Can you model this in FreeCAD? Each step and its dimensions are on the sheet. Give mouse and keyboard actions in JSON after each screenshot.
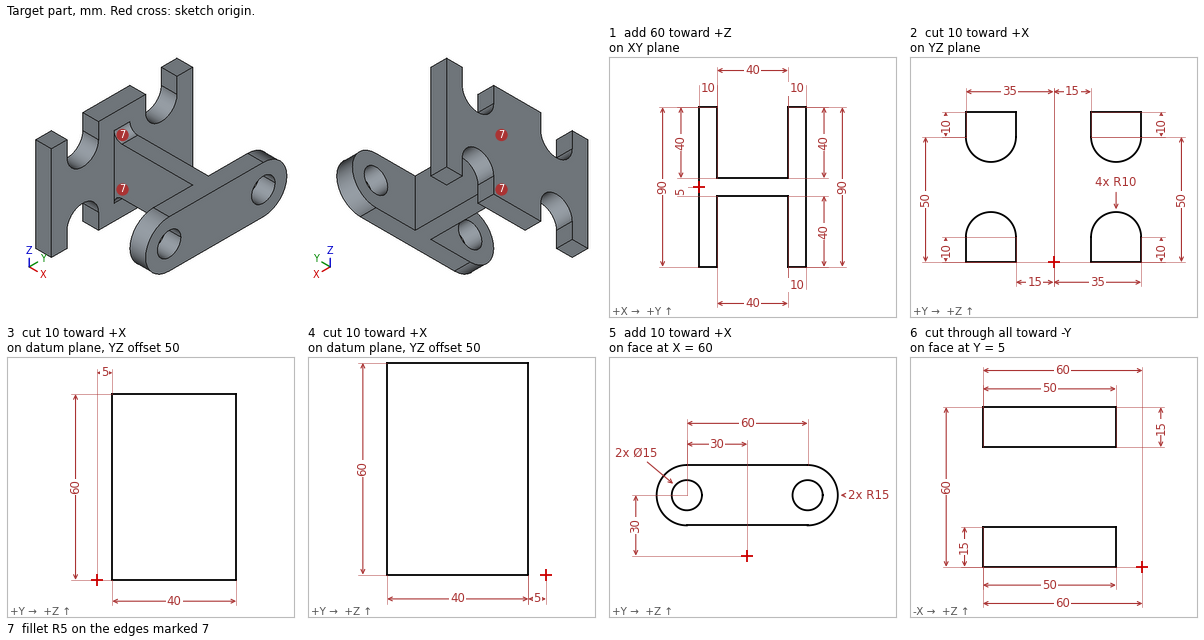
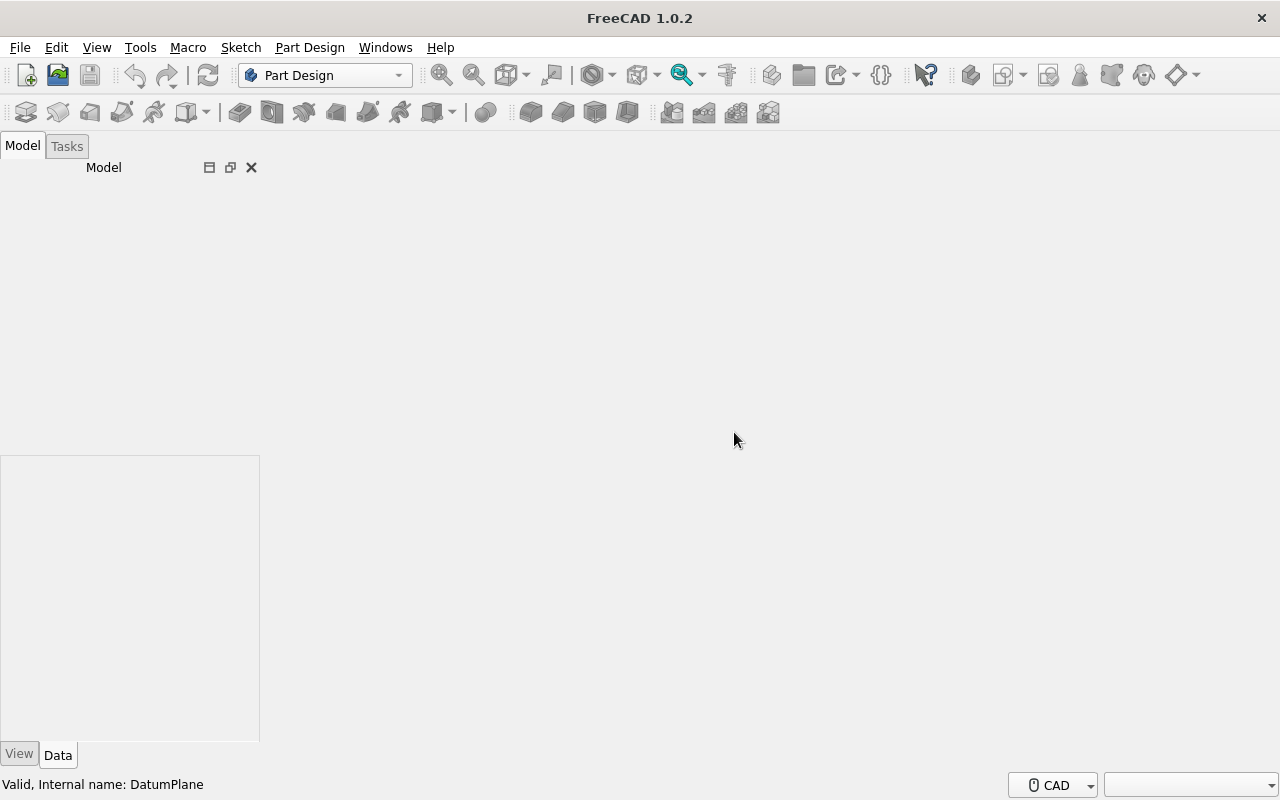
{"action": "left_click", "coordinate": [26, 76]}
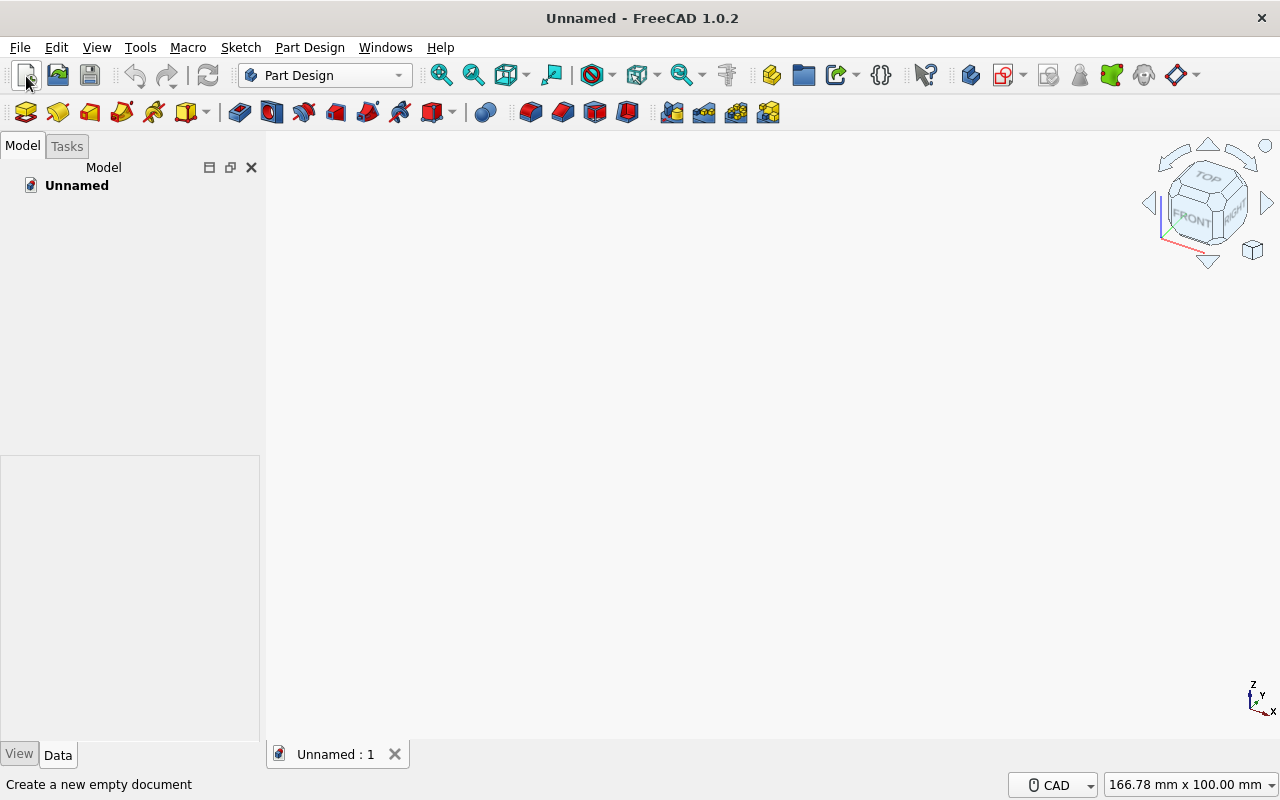
{"action": "left_click", "coordinate": [1004, 76]}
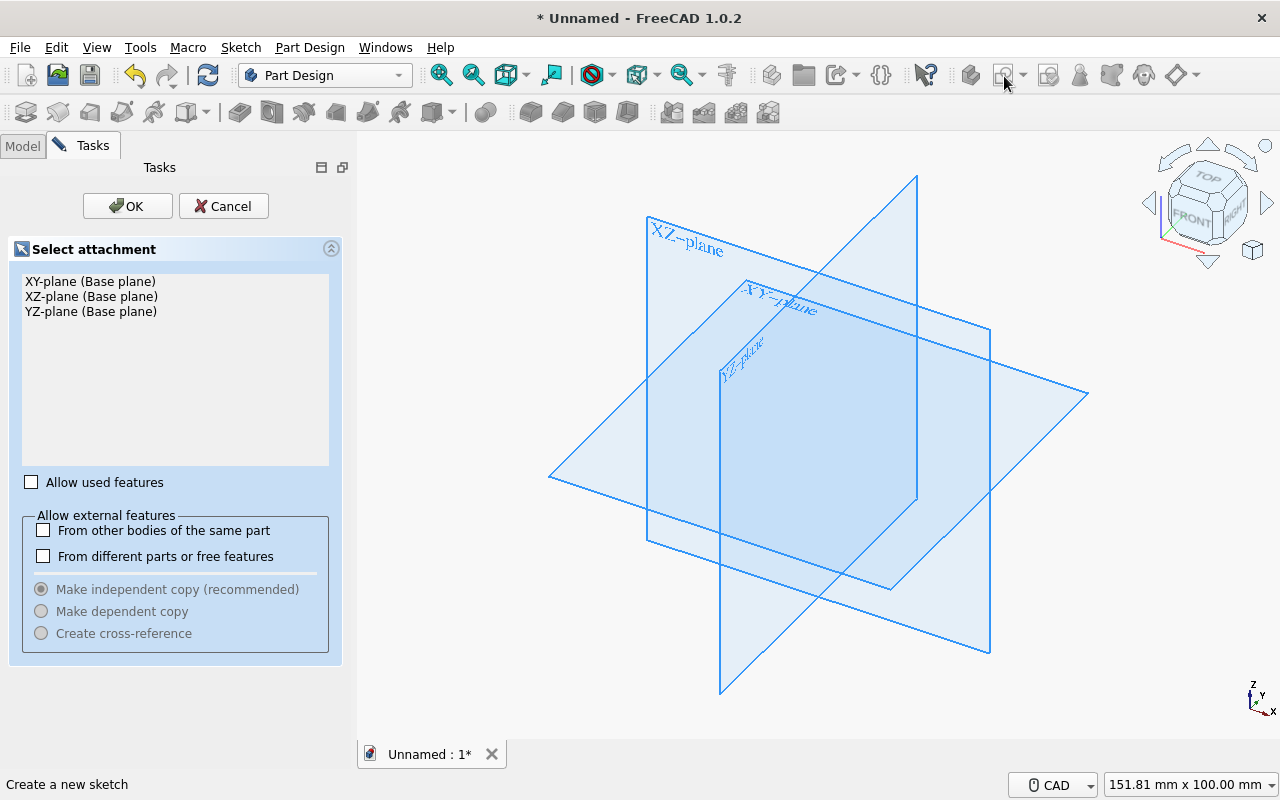
{"action": "left_click", "coordinate": [82, 282]}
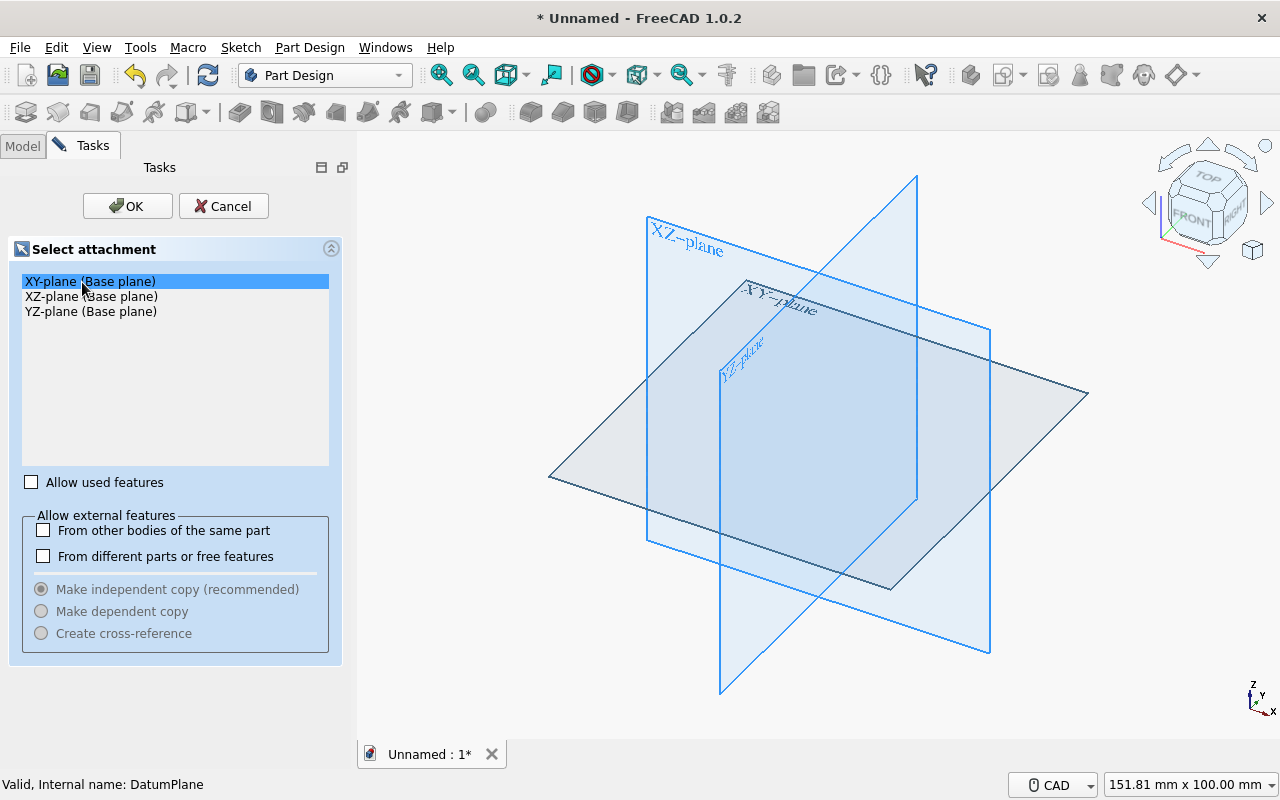
{"action": "left_click", "coordinate": [128, 206]}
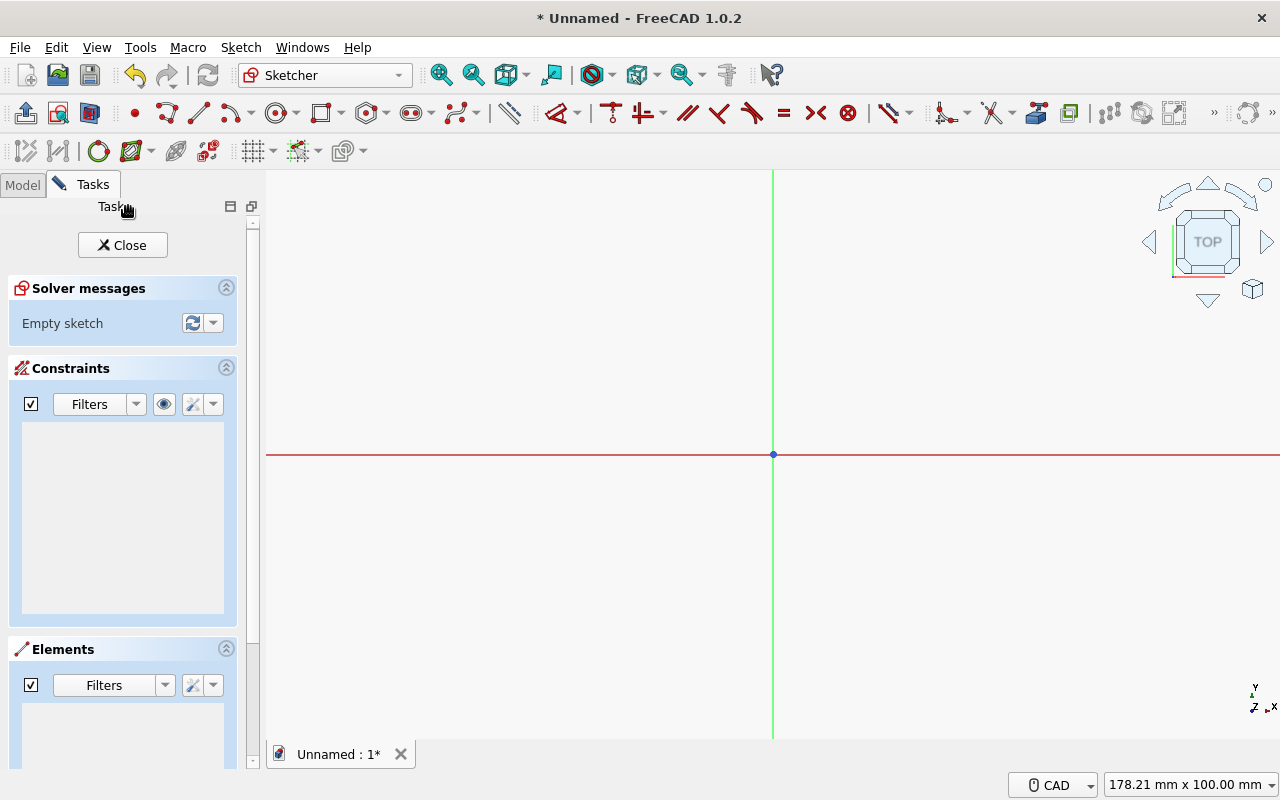
{"action": "scroll", "coordinate": [294, 455], "scroll_direction": "down", "scroll_amount": 2}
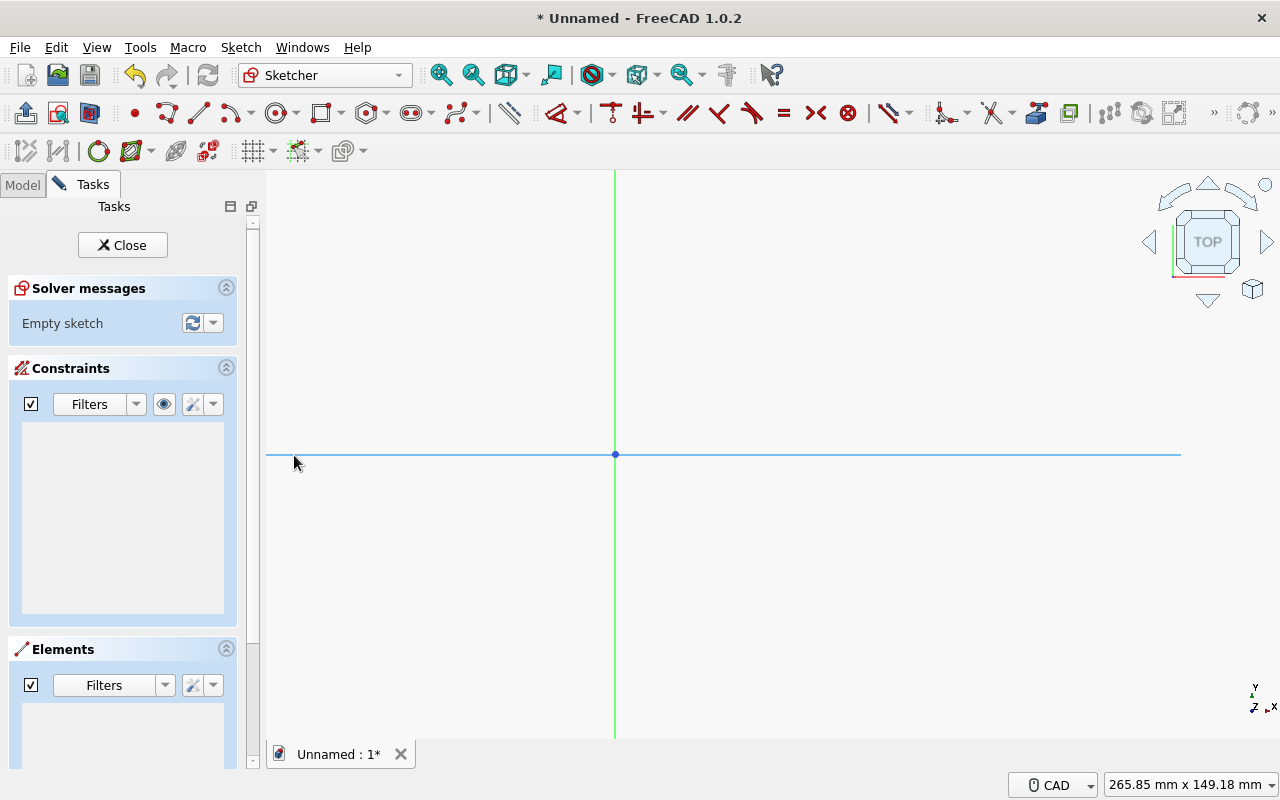
{"action": "left_click", "coordinate": [168, 114]}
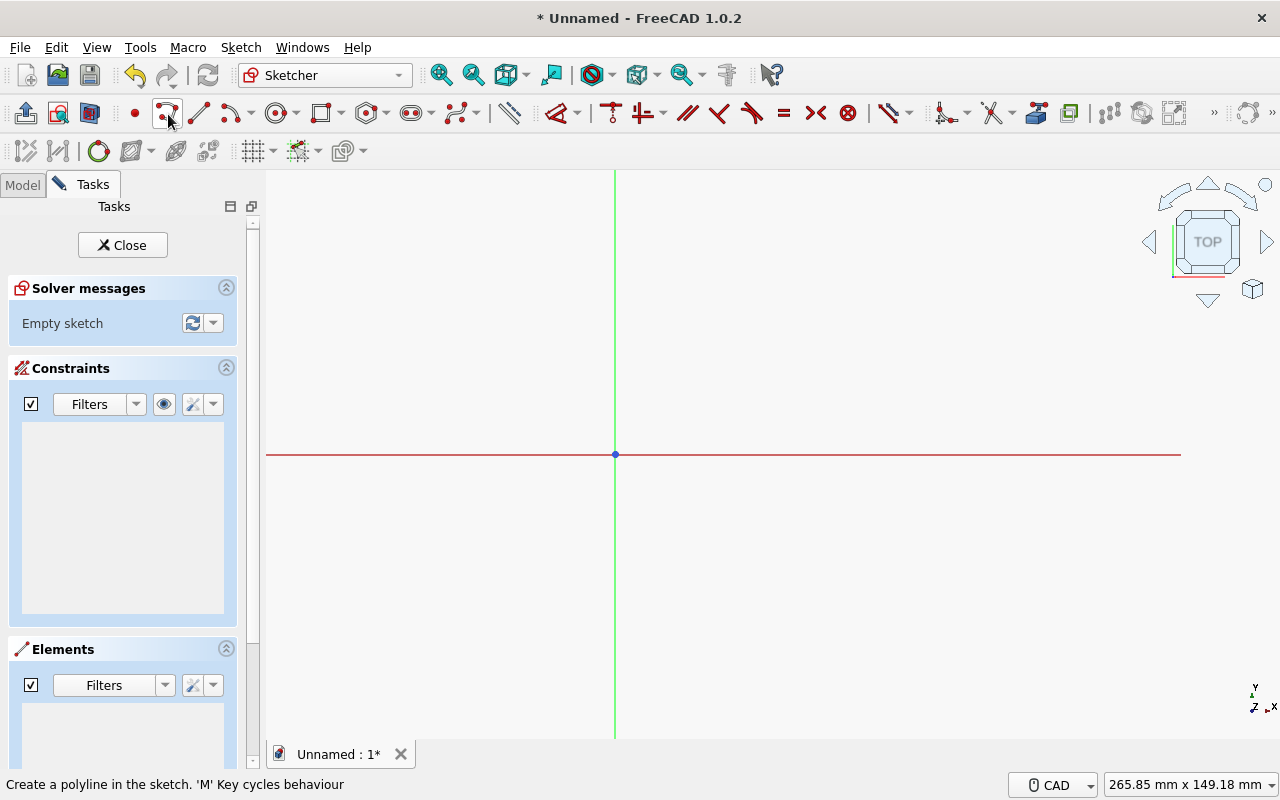
{"action": "left_click", "coordinate": [653, 474]}
{"action": "left_click", "coordinate": [806, 474]}
{"action": "left_click", "coordinate": [806, 626]}
{"action": "left_click", "coordinate": [844, 626]}
{"action": "left_click", "coordinate": [844, 283]}
{"action": "left_click", "coordinate": [806, 283]}
{"action": "left_click", "coordinate": [806, 436]}
{"action": "left_click", "coordinate": [653, 436]}
{"action": "left_click", "coordinate": [653, 283]}
{"action": "left_click", "coordinate": [615, 283]}
{"action": "left_click", "coordinate": [624, 626]}
{"action": "left_click", "coordinate": [653, 626]}
{"action": "left_click", "coordinate": [653, 475]}
{"action": "key", "text": "Escape"}
{"action": "key", "text": "Escape"}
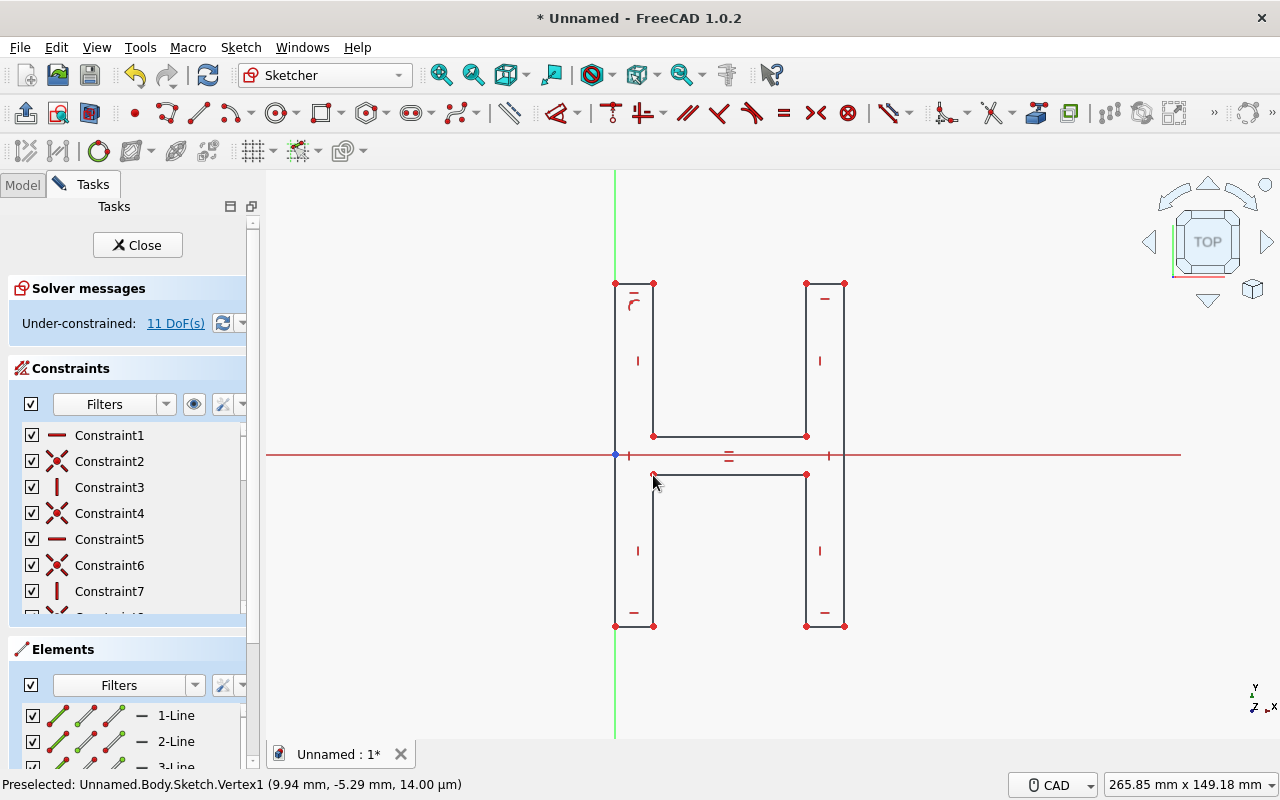
{"action": "left_click", "coordinate": [556, 114]}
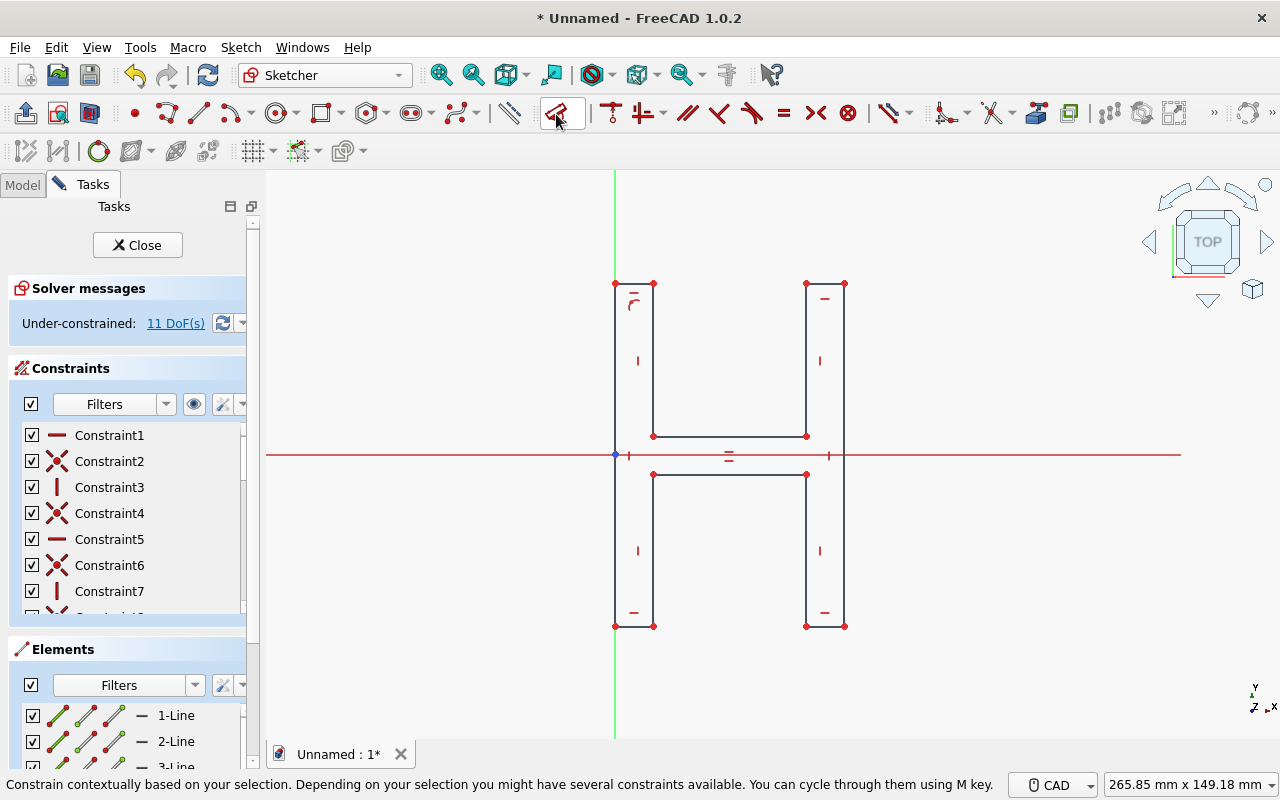
{"action": "left_click", "coordinate": [699, 475]}
{"action": "left_click", "coordinate": [729, 509]}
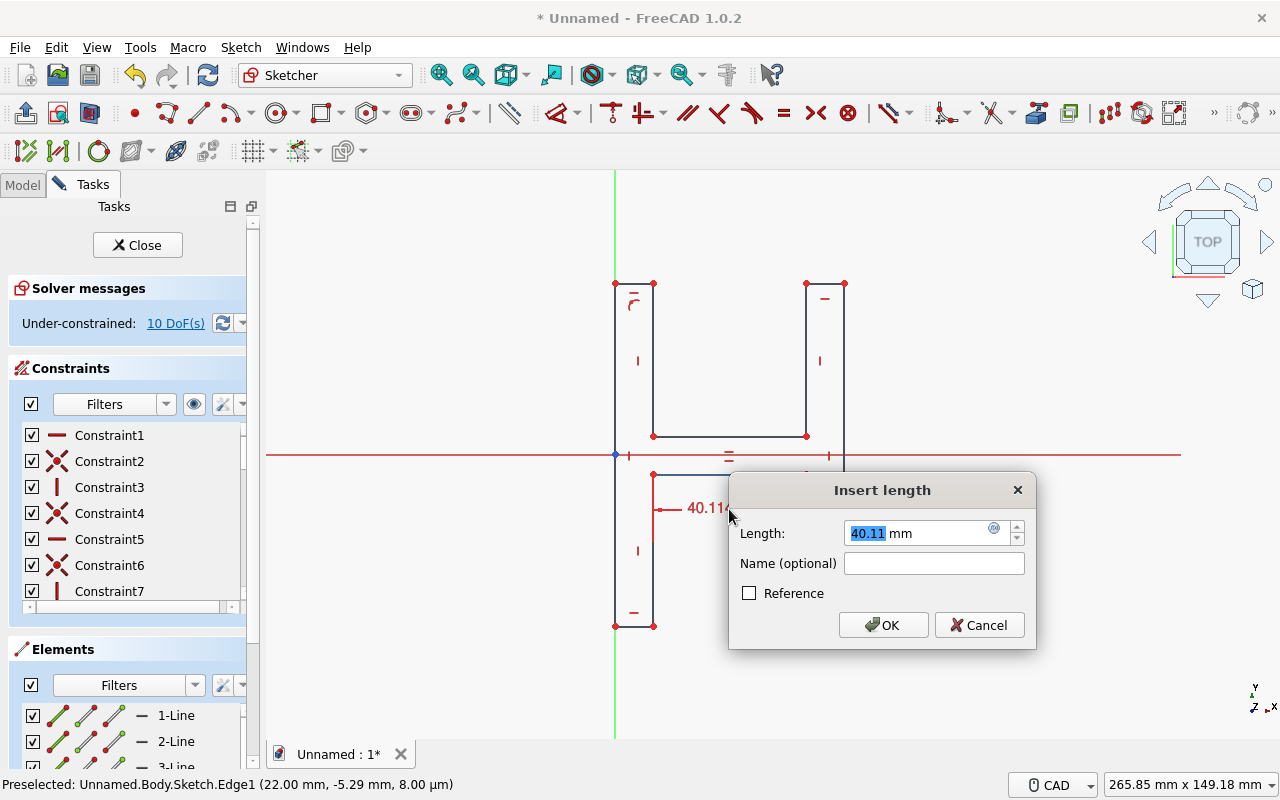
{"action": "type", "text": "40"}
{"action": "key", "text": "Return"}